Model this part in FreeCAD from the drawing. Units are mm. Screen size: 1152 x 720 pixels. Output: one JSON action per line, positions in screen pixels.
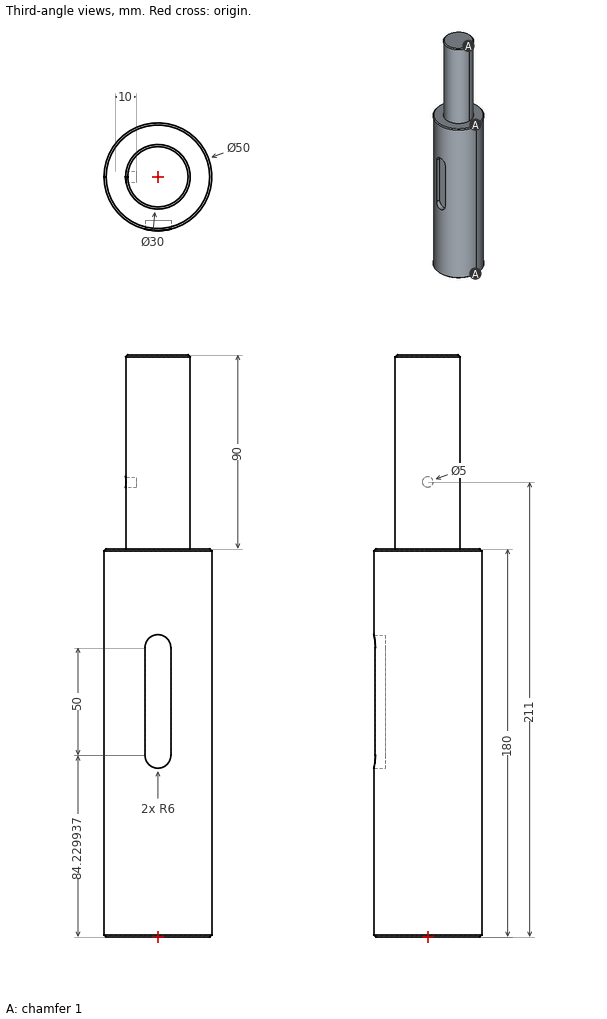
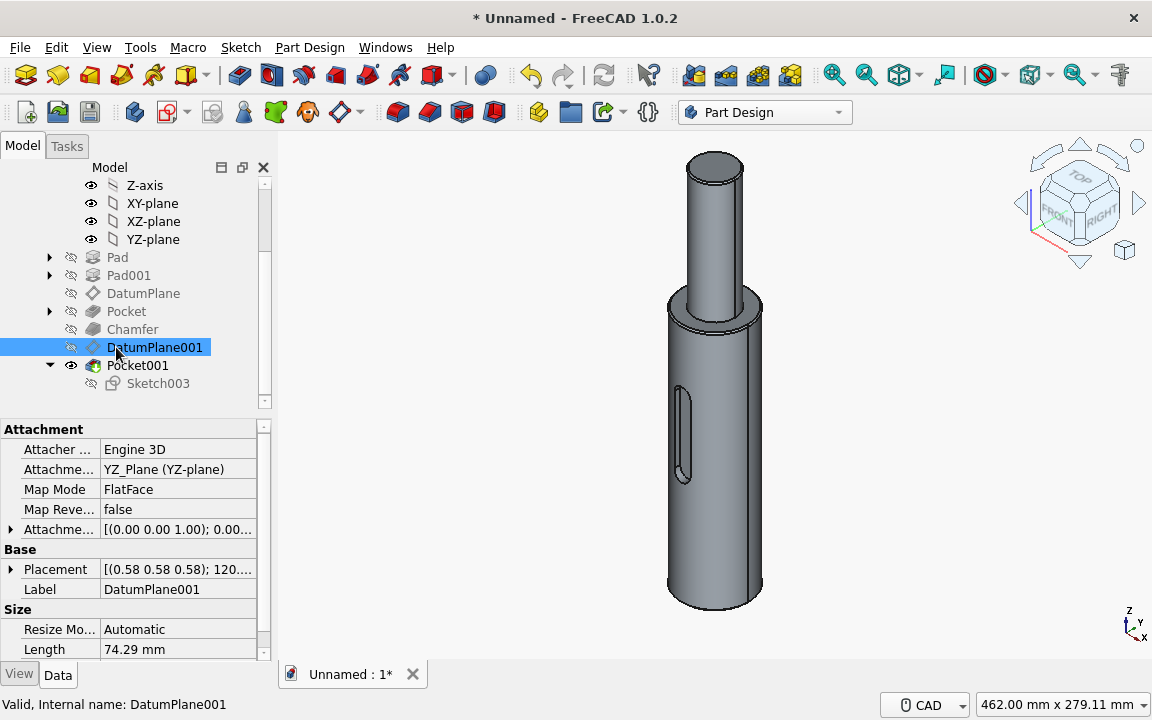
{"action": "left_click", "coordinate": [836, 76]}